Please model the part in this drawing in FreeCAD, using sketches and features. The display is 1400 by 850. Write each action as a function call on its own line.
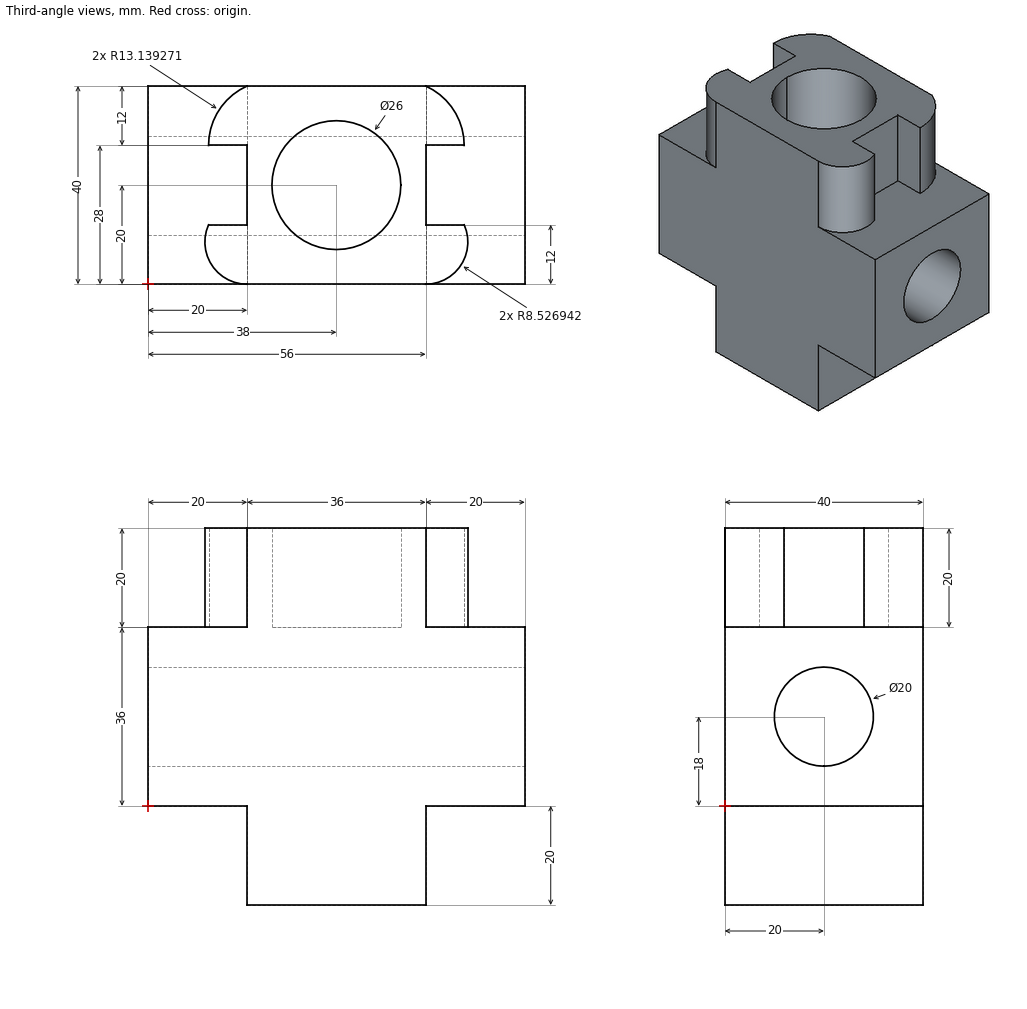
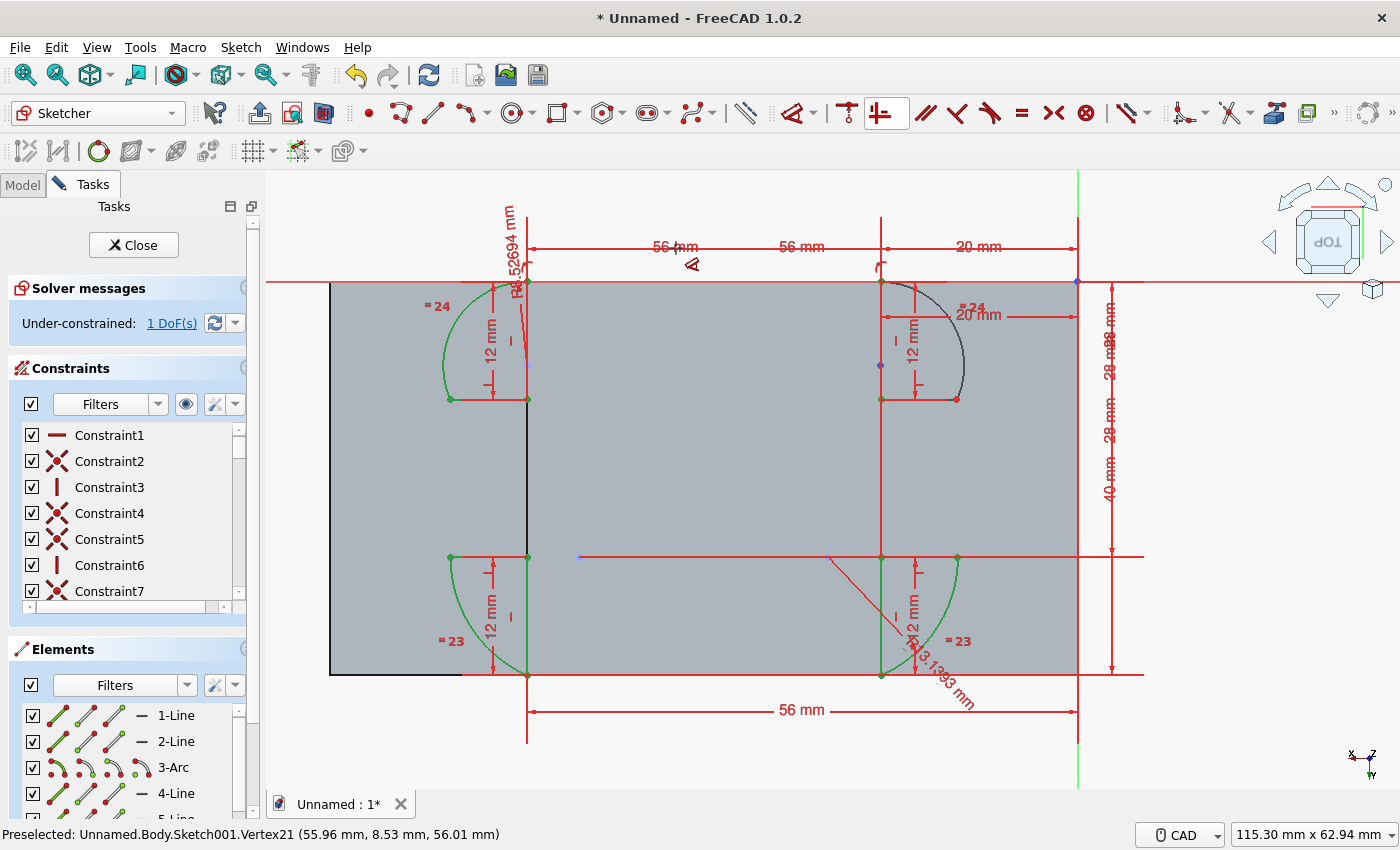
click(880, 366)
click(979, 400)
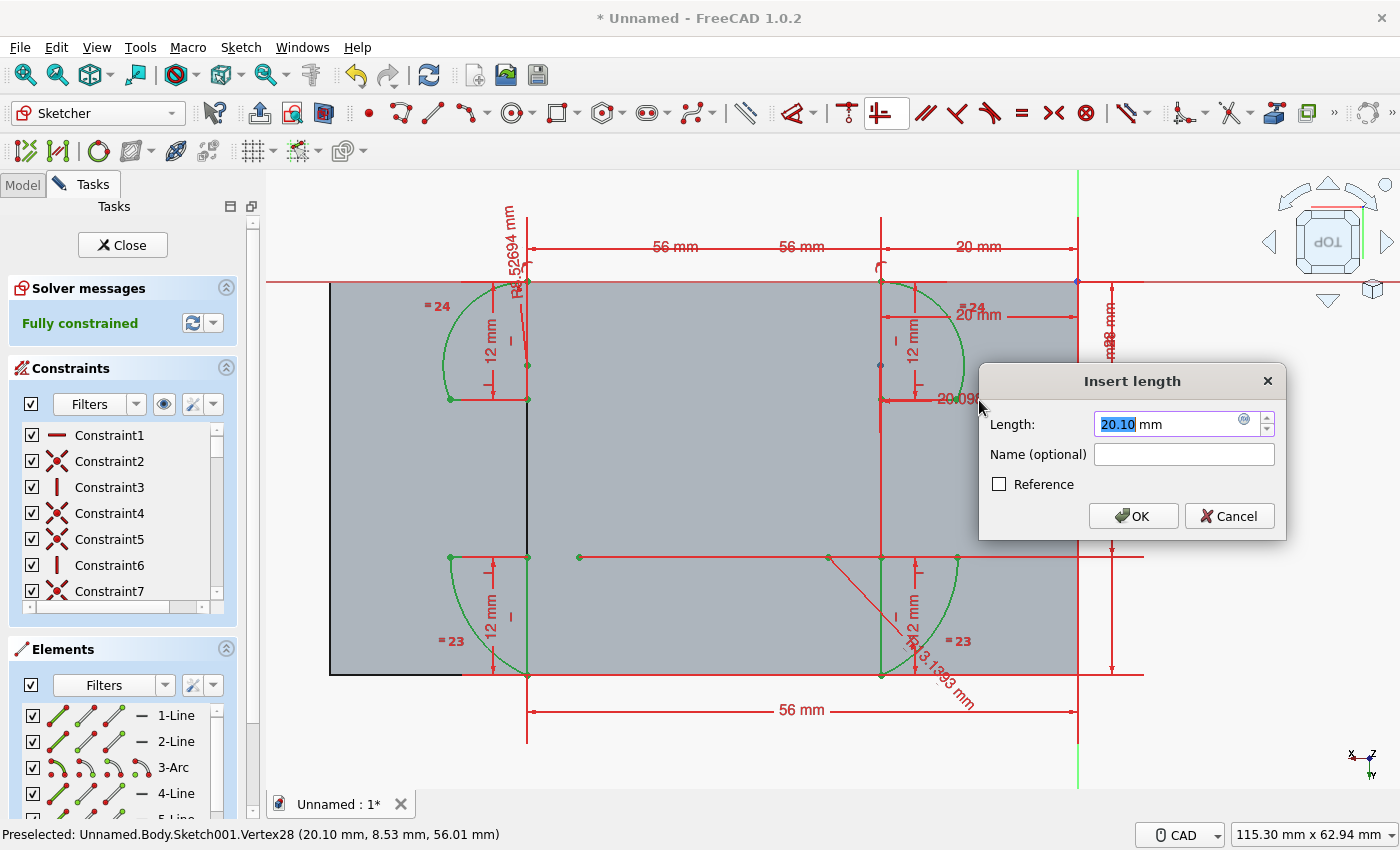
text(20)
key(Return)
key(Escape)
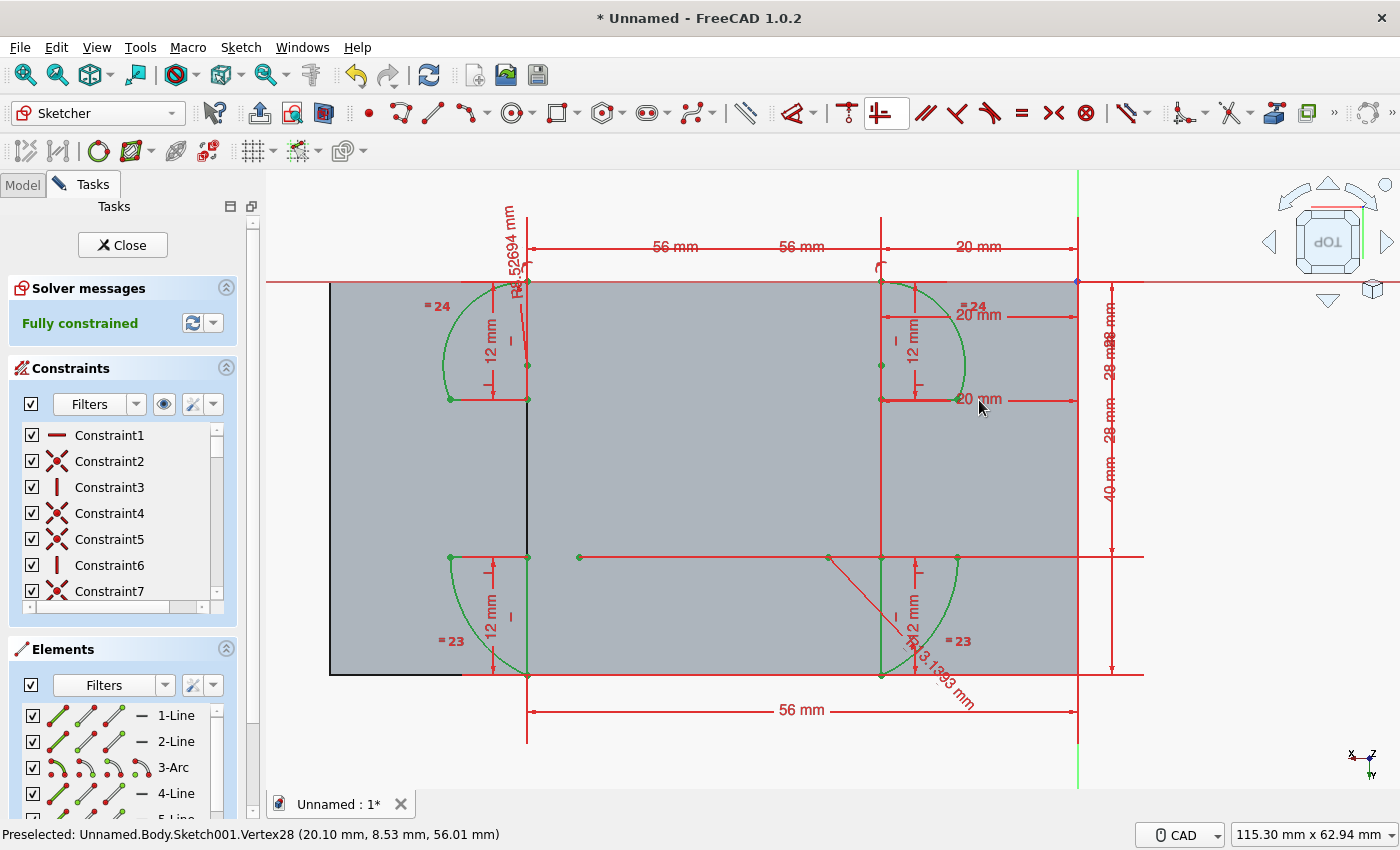
click(123, 245)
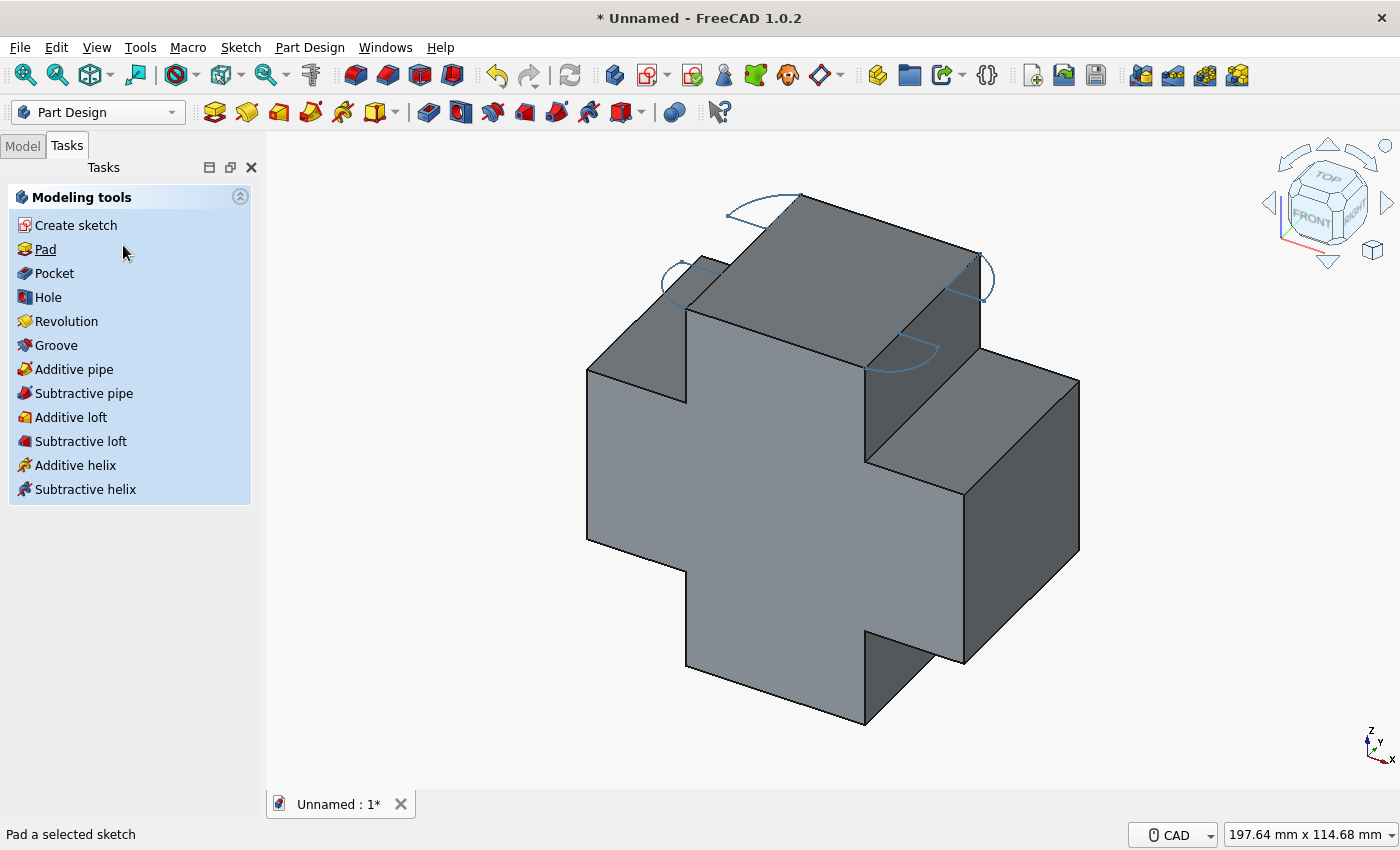
click(216, 112)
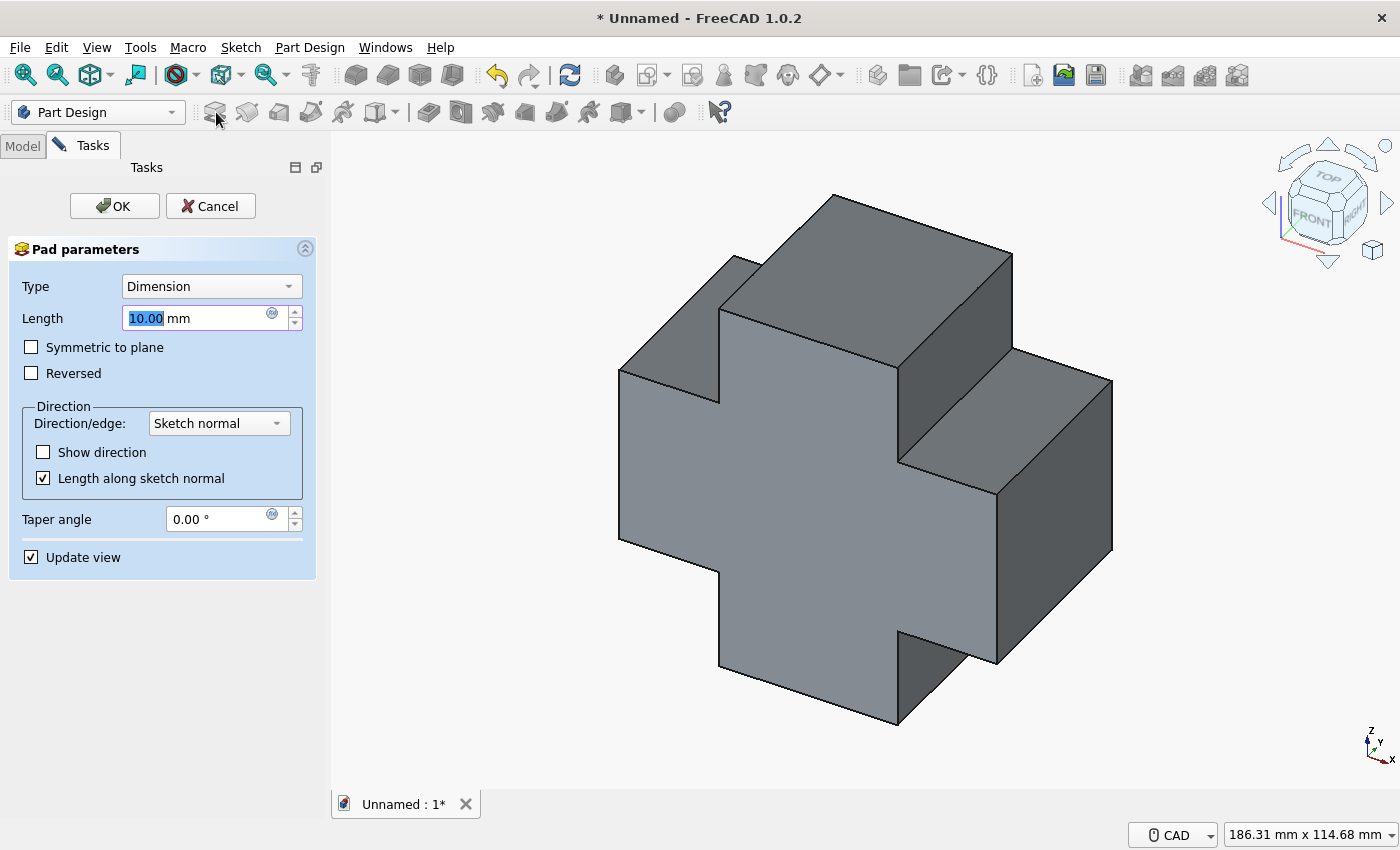
text(20)
key(Tab)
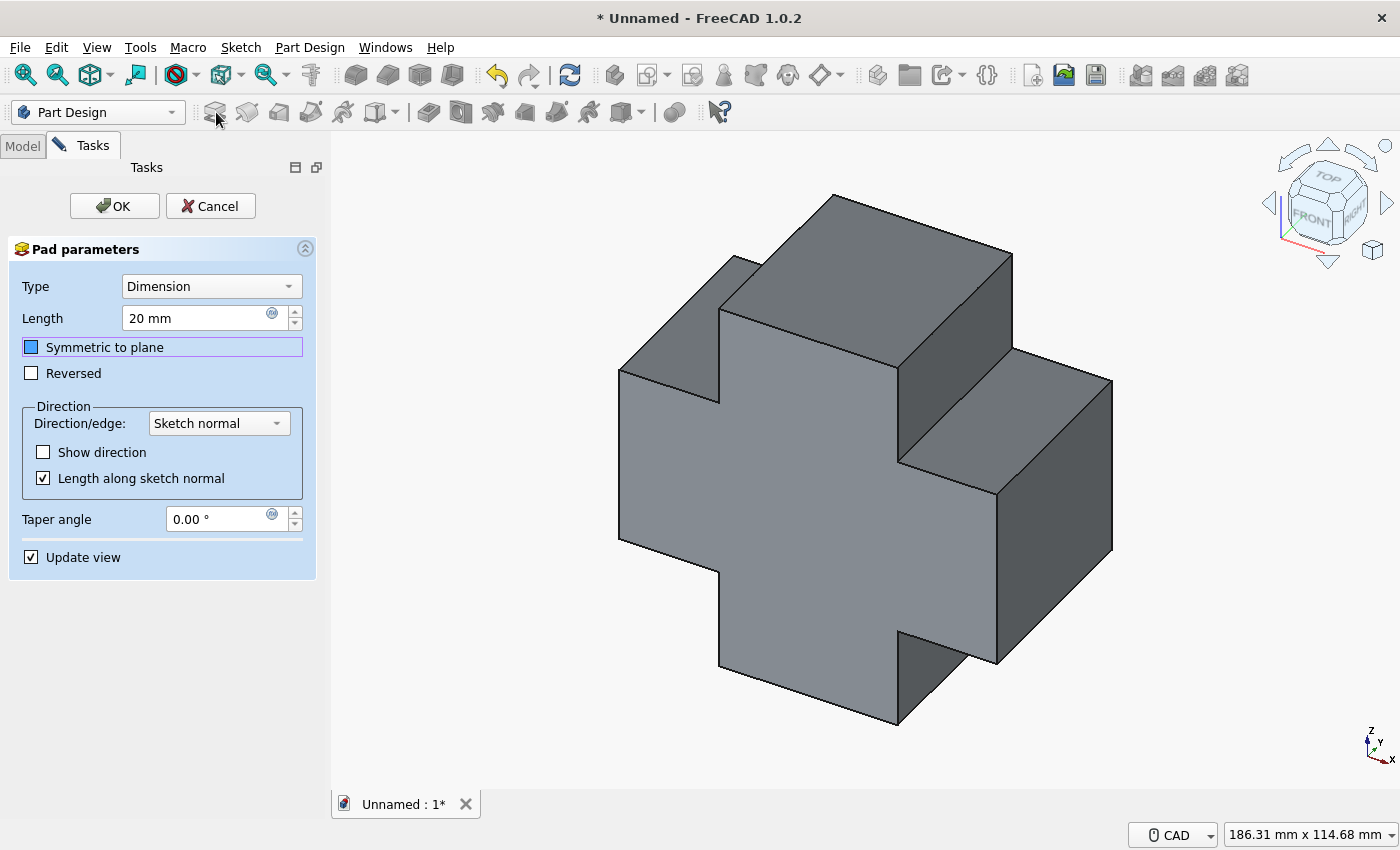
click(30, 373)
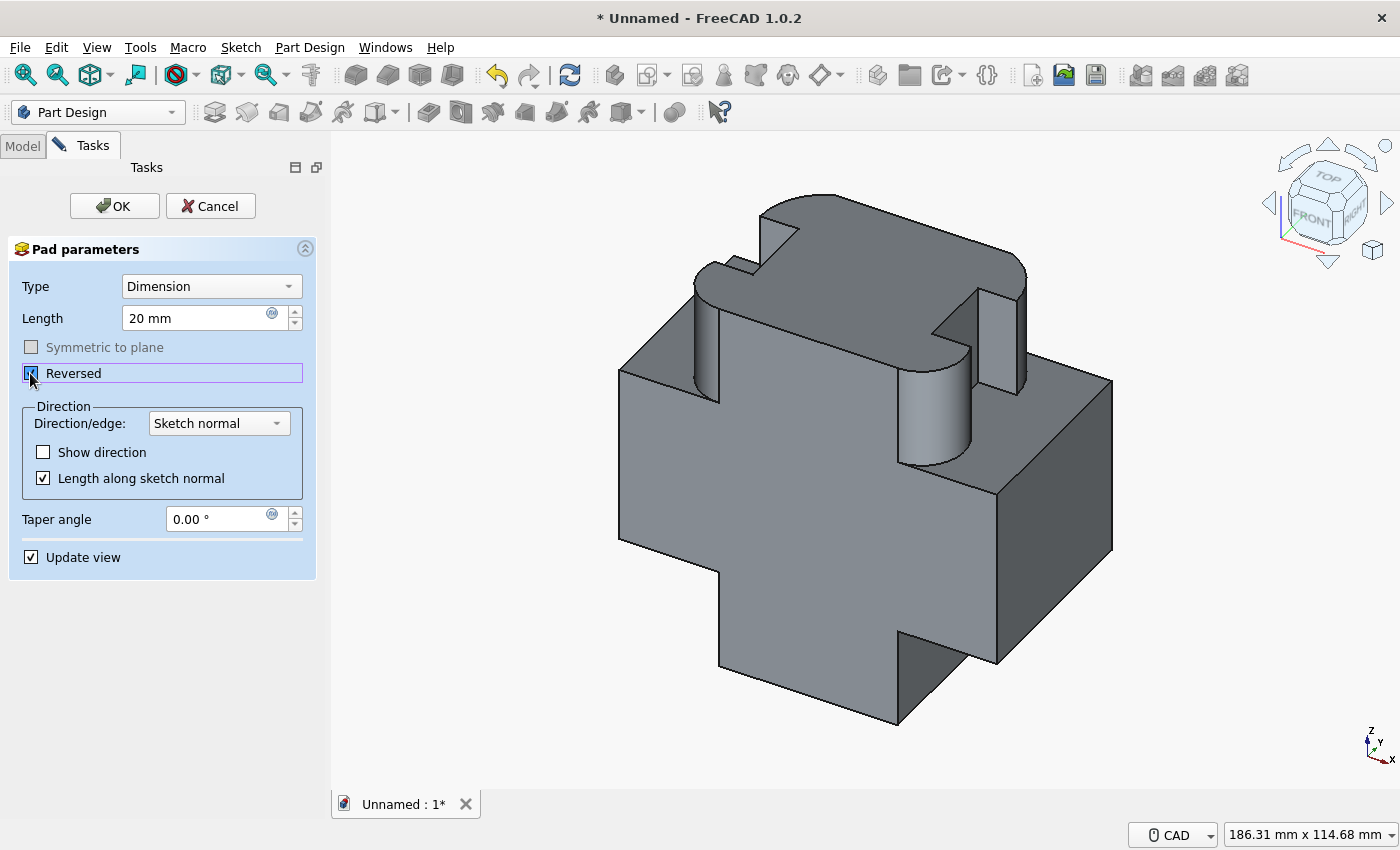
click(115, 206)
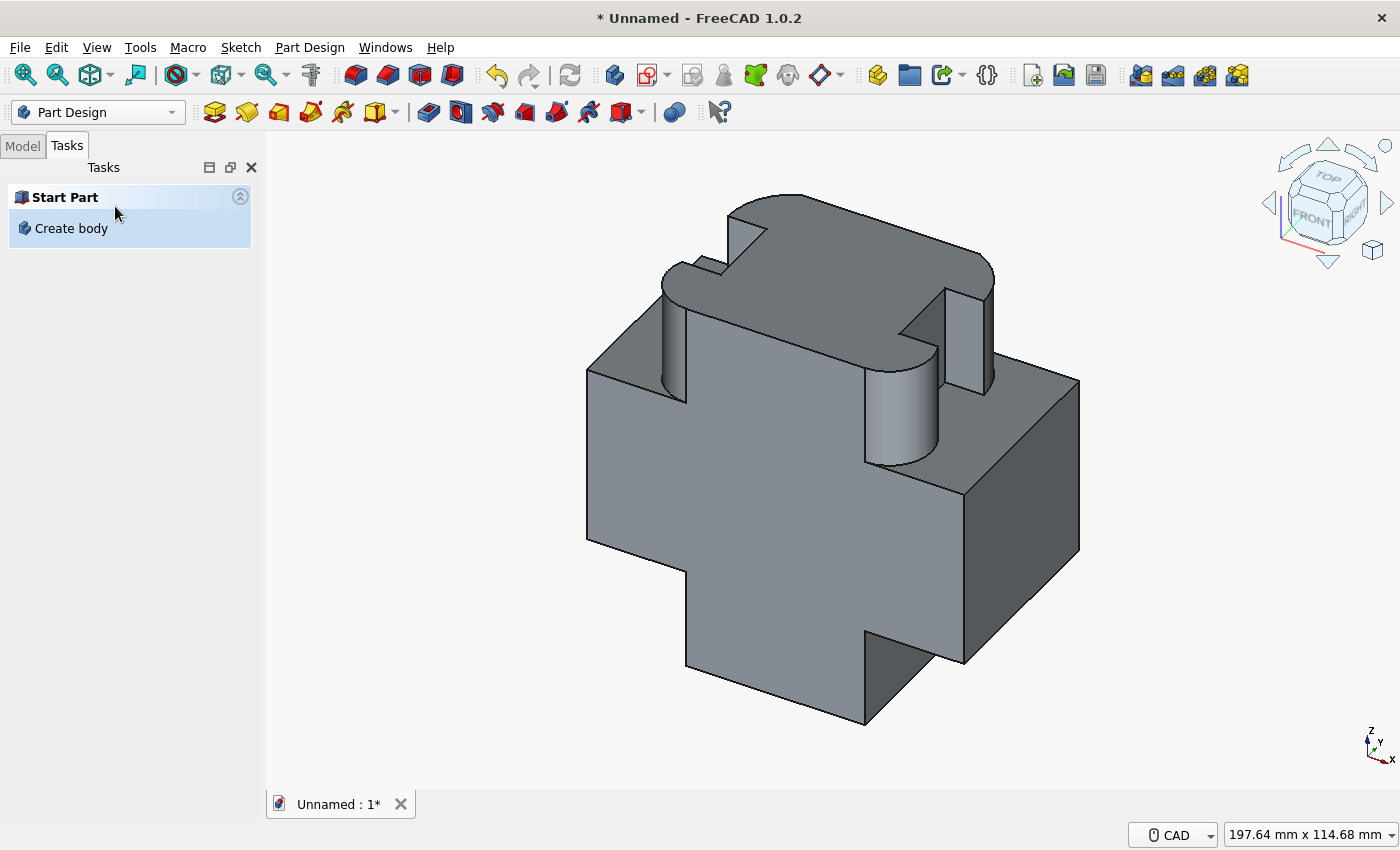
click(833, 280)